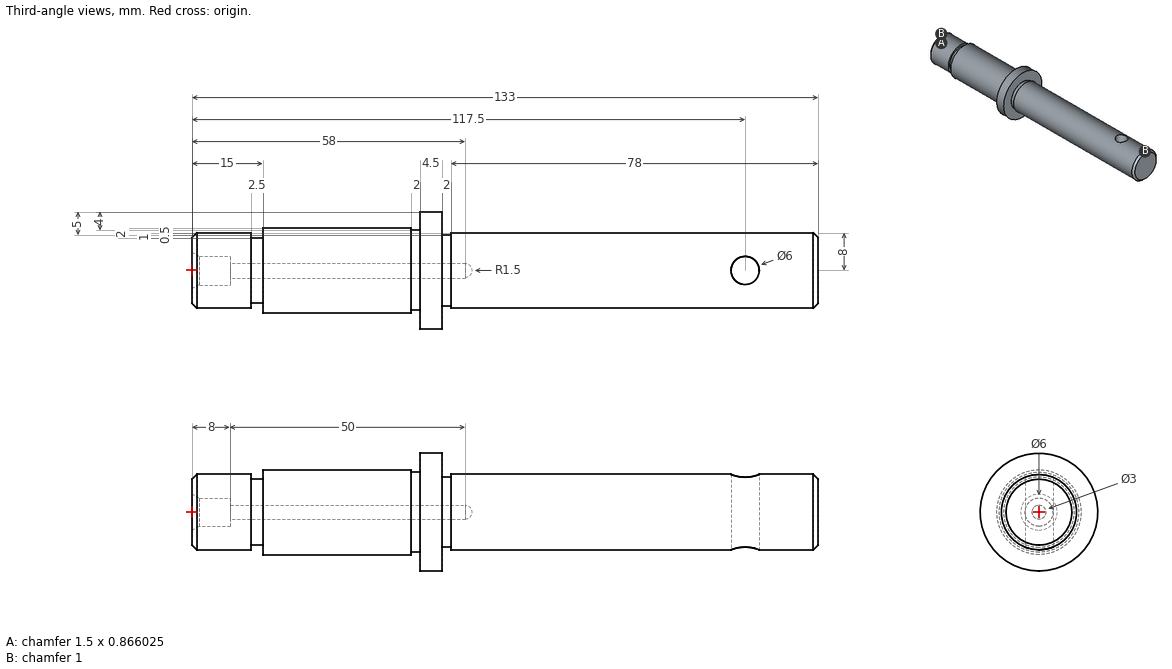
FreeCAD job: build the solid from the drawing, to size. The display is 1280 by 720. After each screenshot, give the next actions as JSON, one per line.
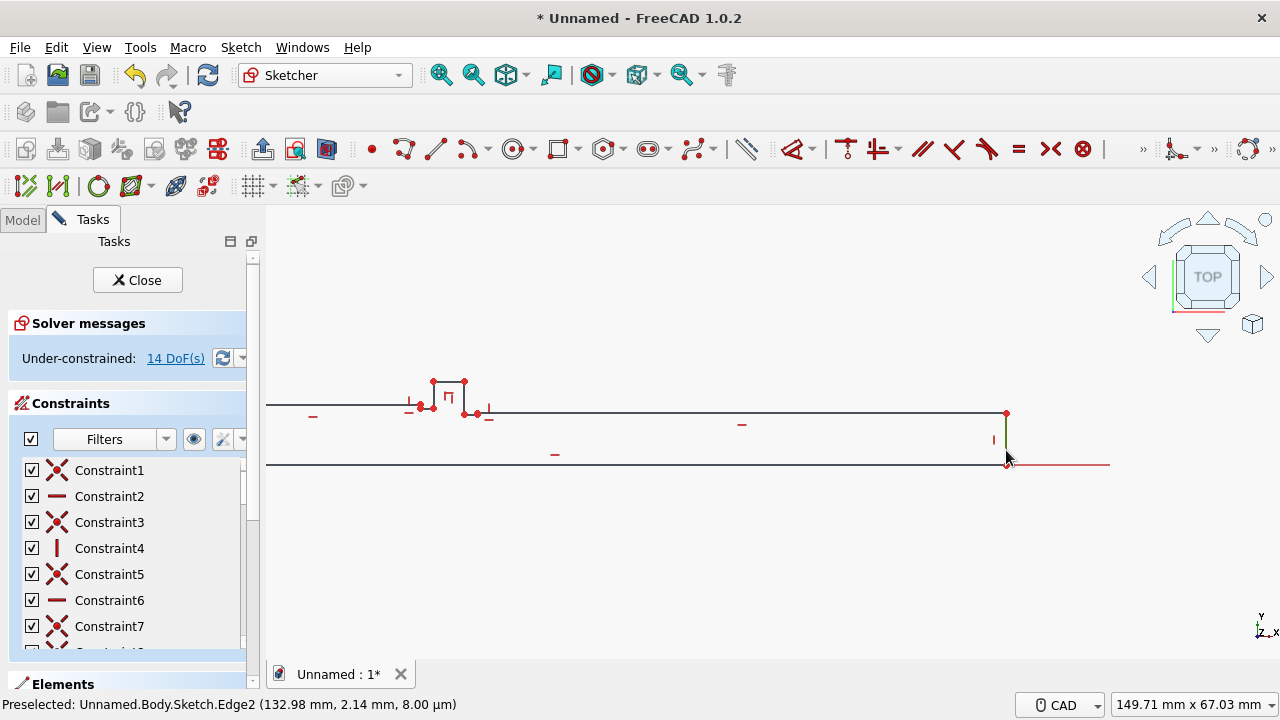
{"action": "left_click", "coordinate": [814, 150]}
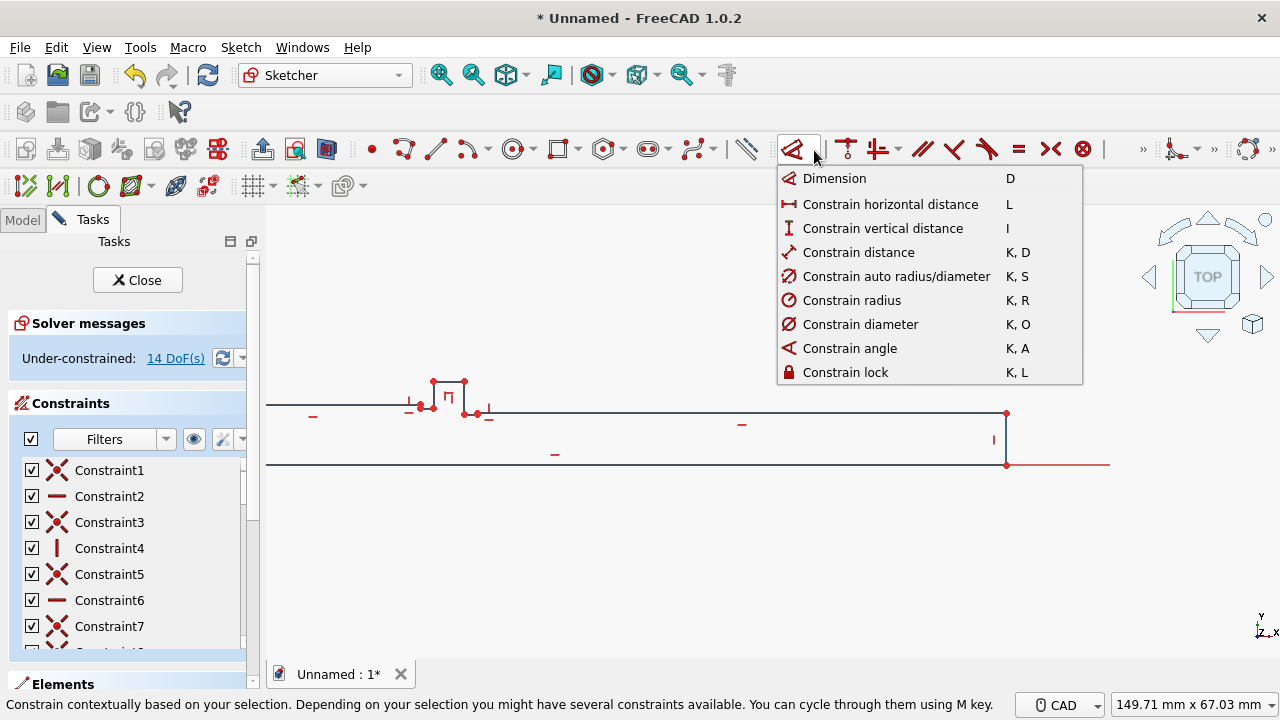
{"action": "left_click", "coordinate": [930, 228]}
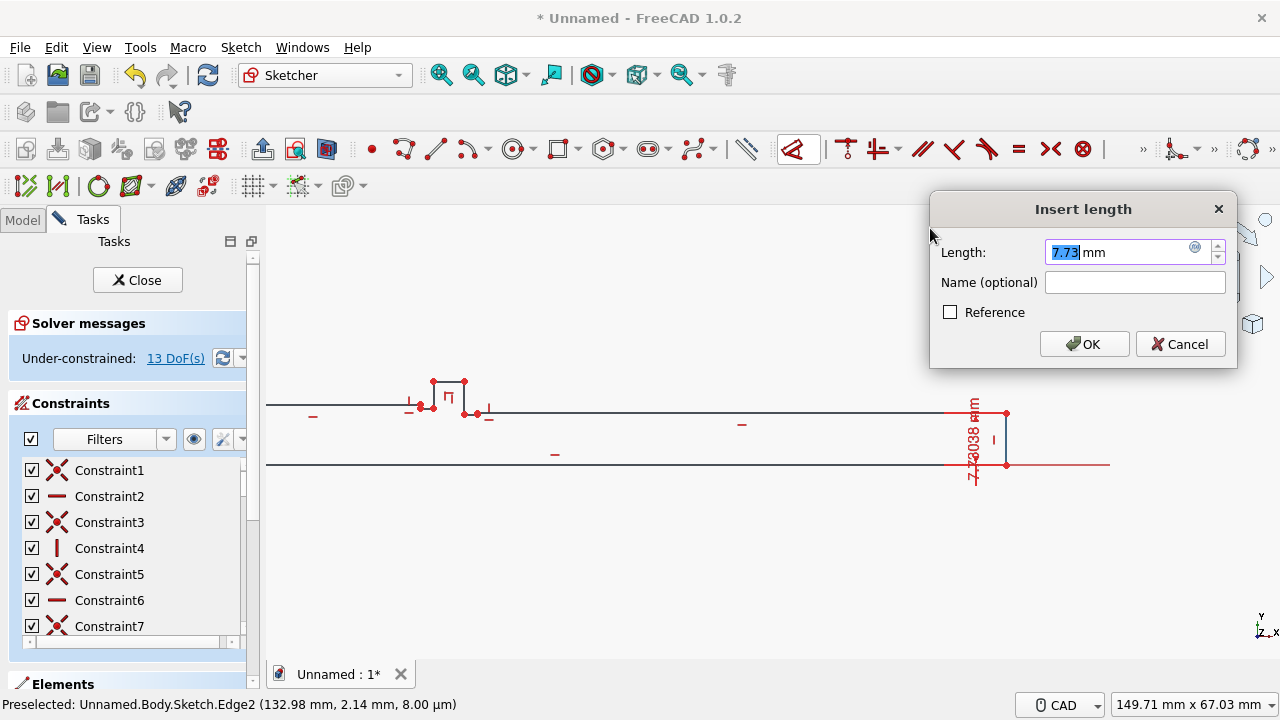
{"action": "type", "text": "8"}
{"action": "key", "text": "Return"}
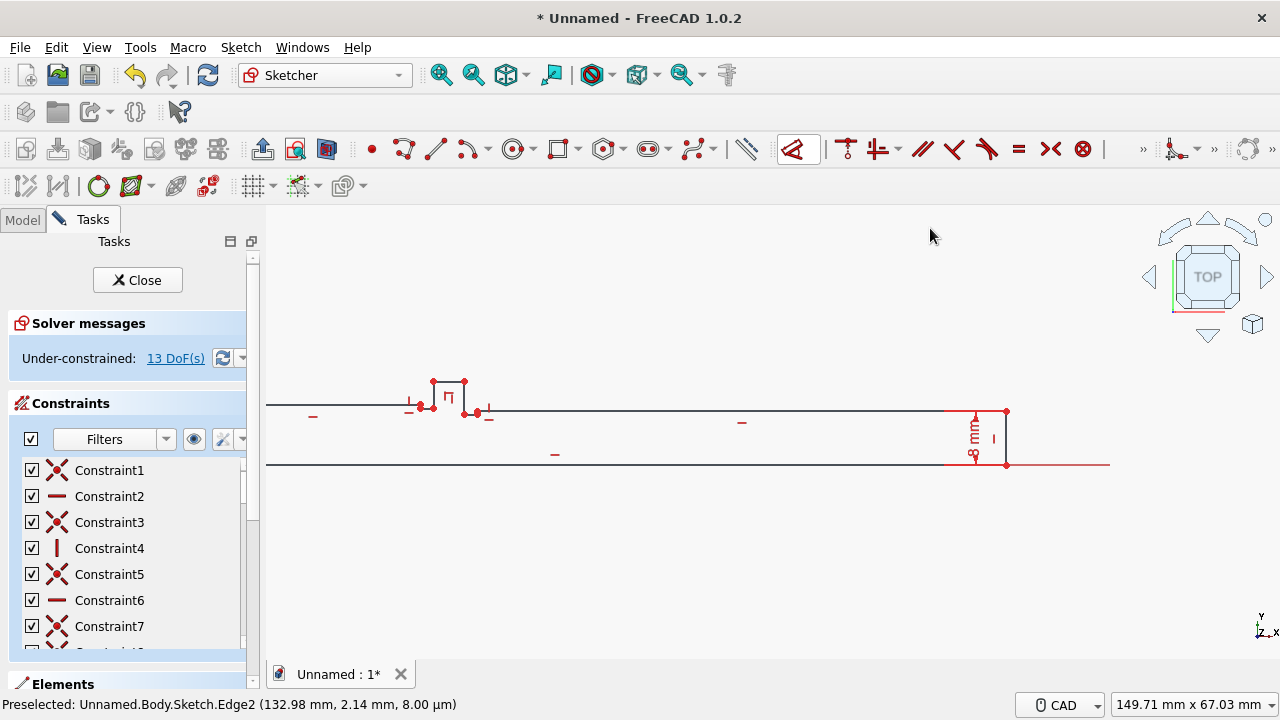
{"action": "scroll", "coordinate": [471, 415], "scroll_direction": "up", "scroll_amount": 6}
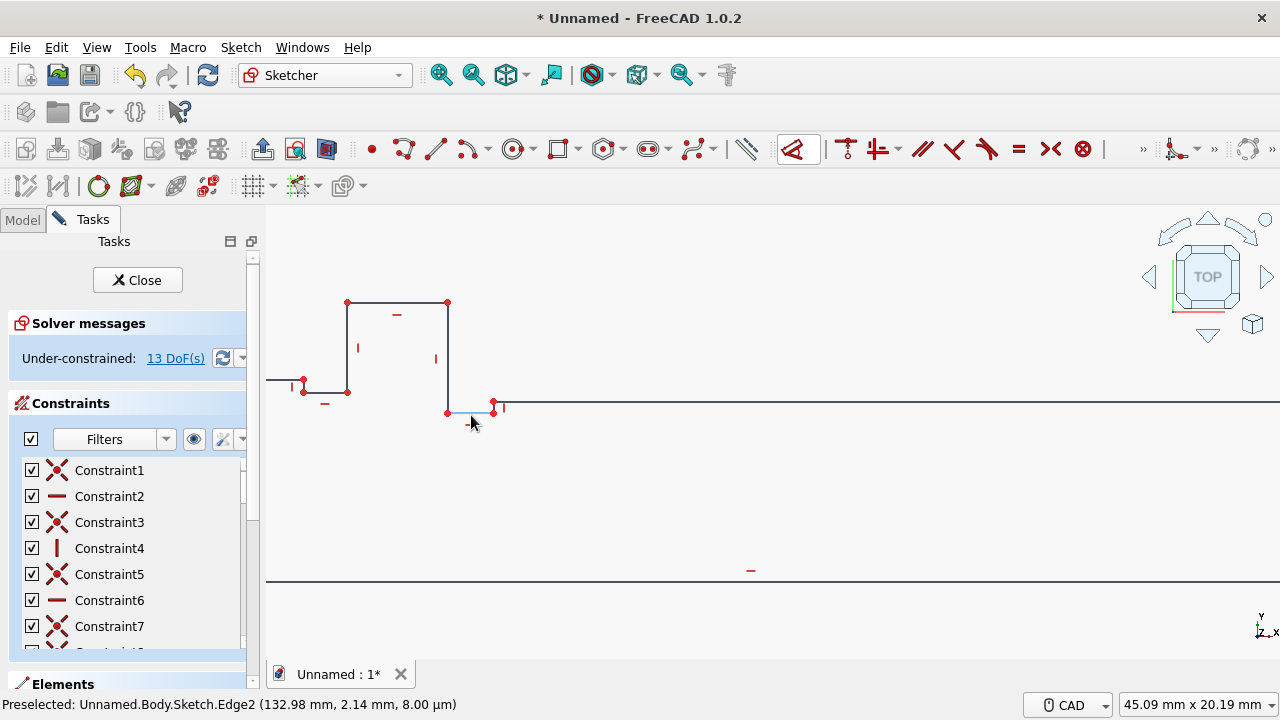
{"action": "left_click", "coordinate": [471, 413]}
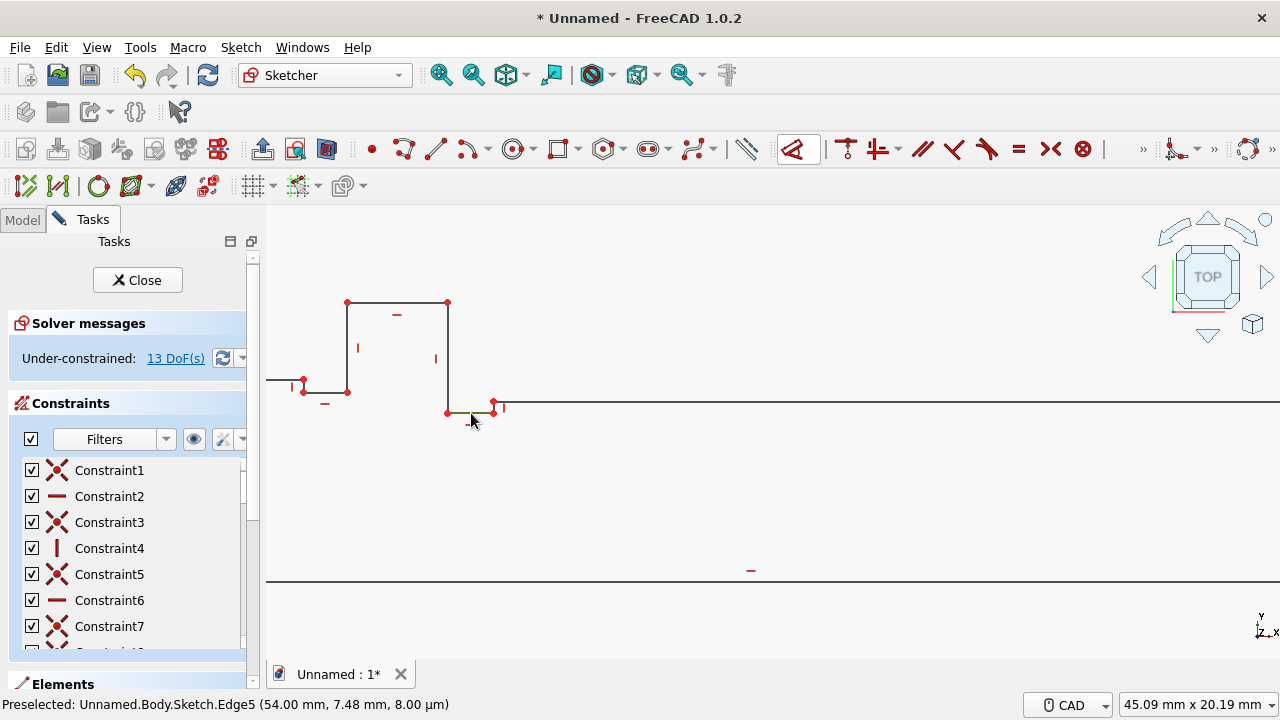
{"action": "key", "text": "l"}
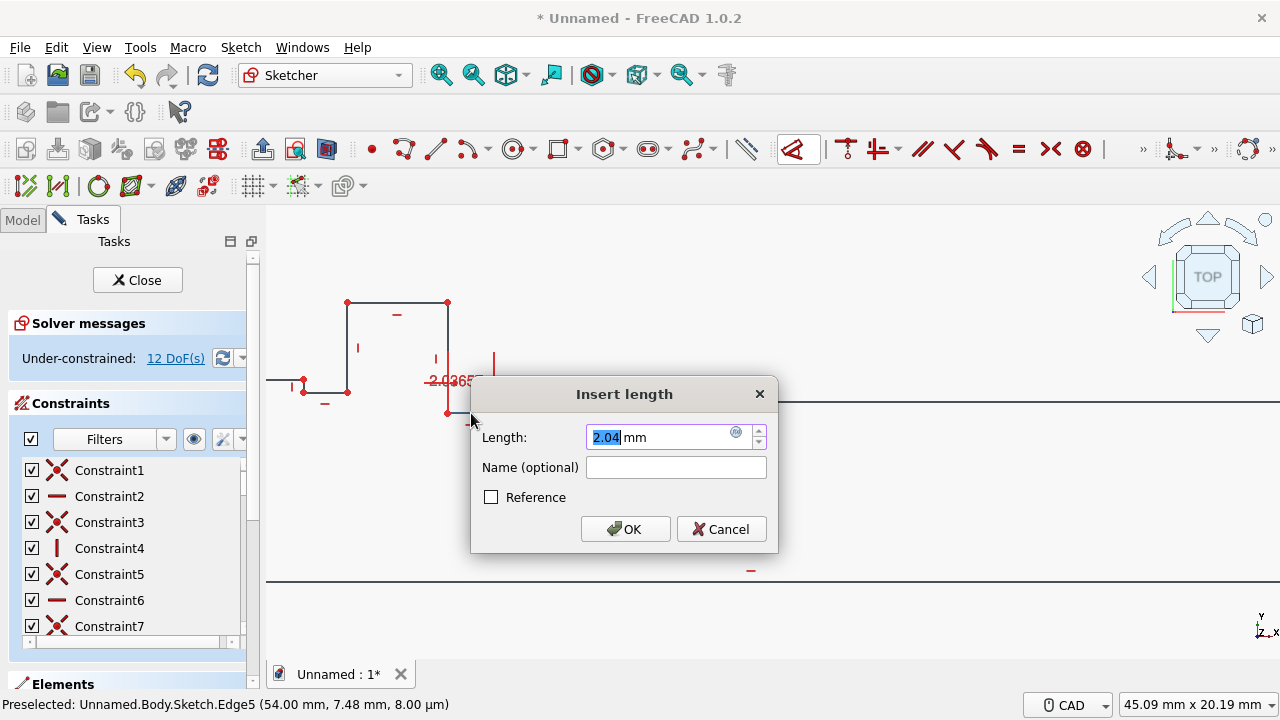
{"action": "type", "text": "2"}
{"action": "key", "text": "Return"}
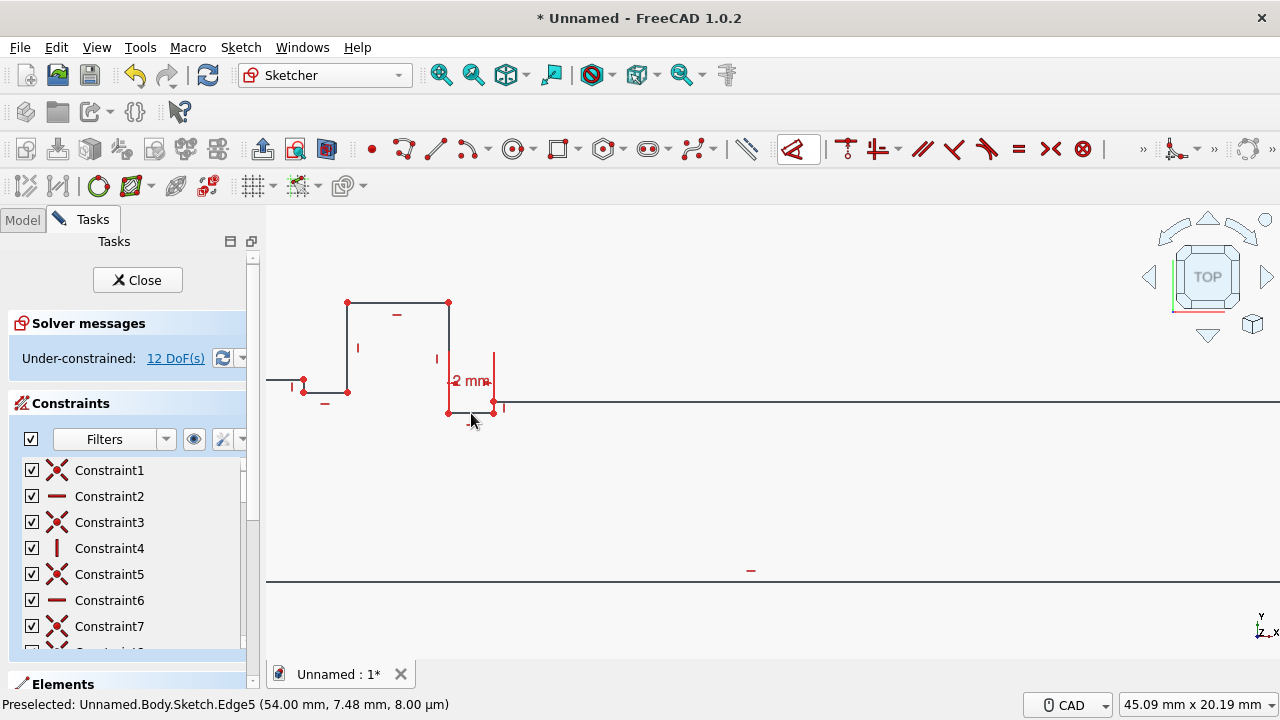
{"action": "left_click", "coordinate": [449, 380]}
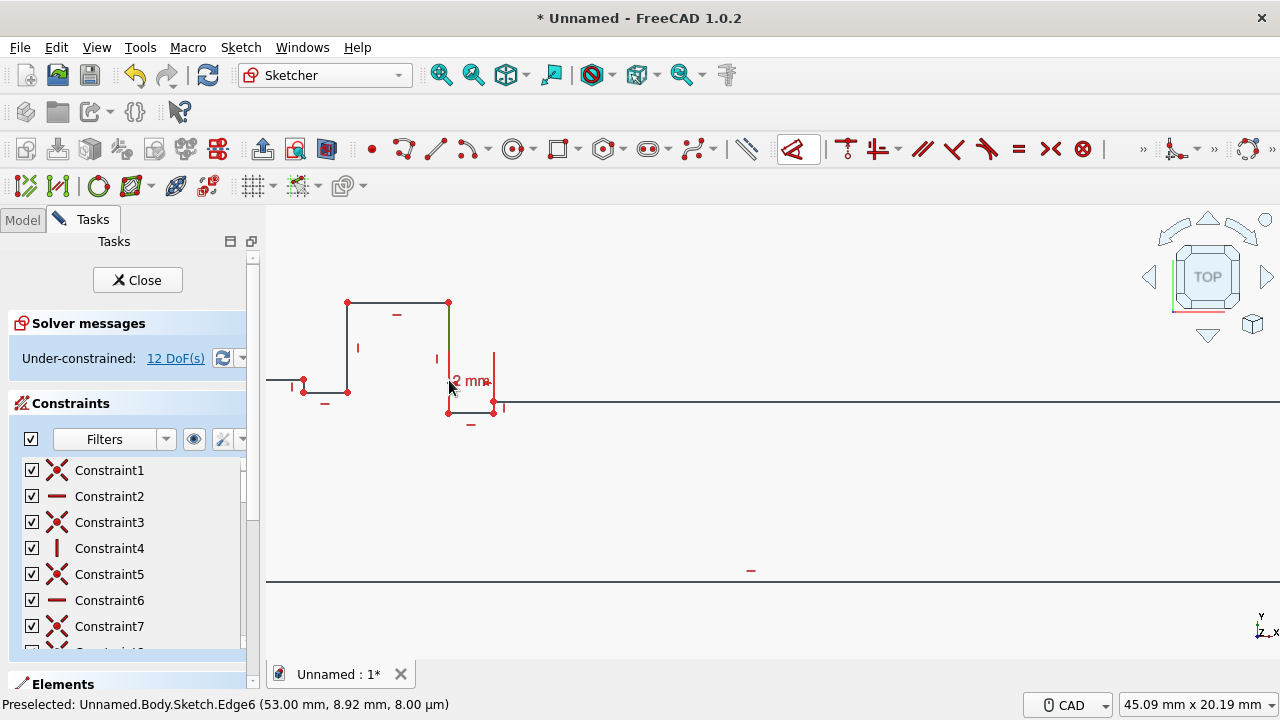
{"action": "left_click", "coordinate": [814, 150]}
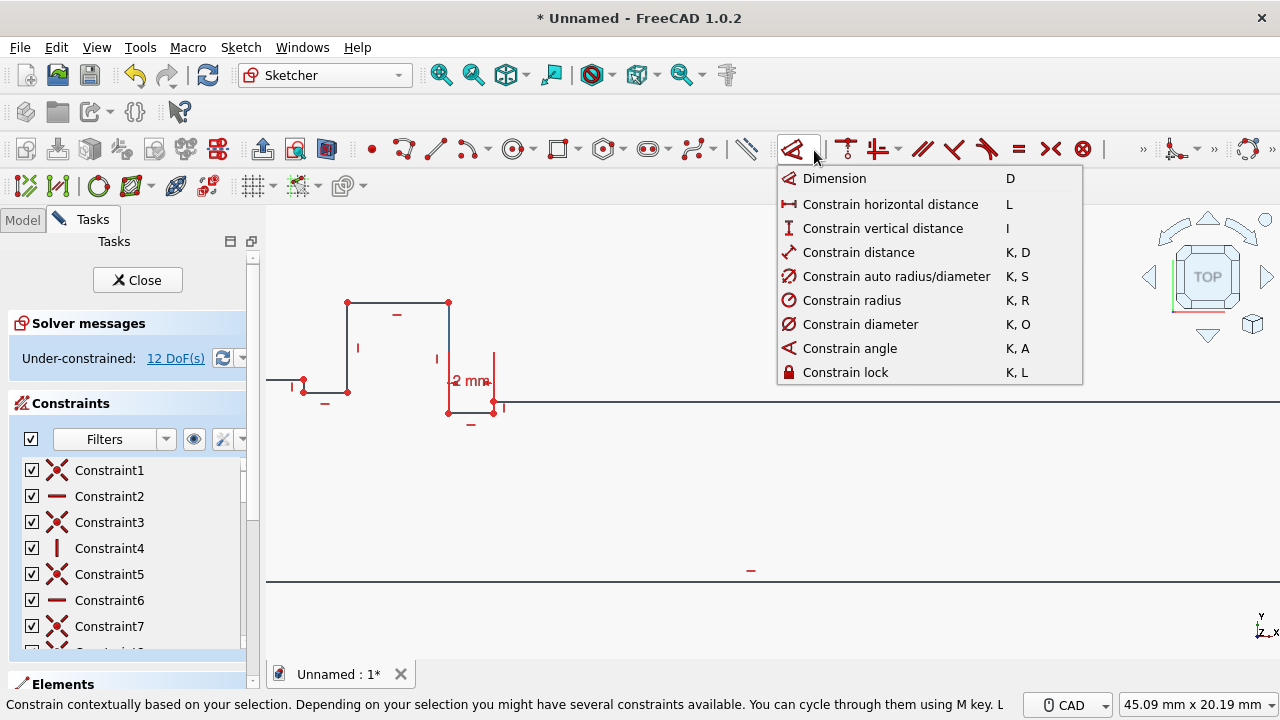
{"action": "left_click", "coordinate": [930, 228]}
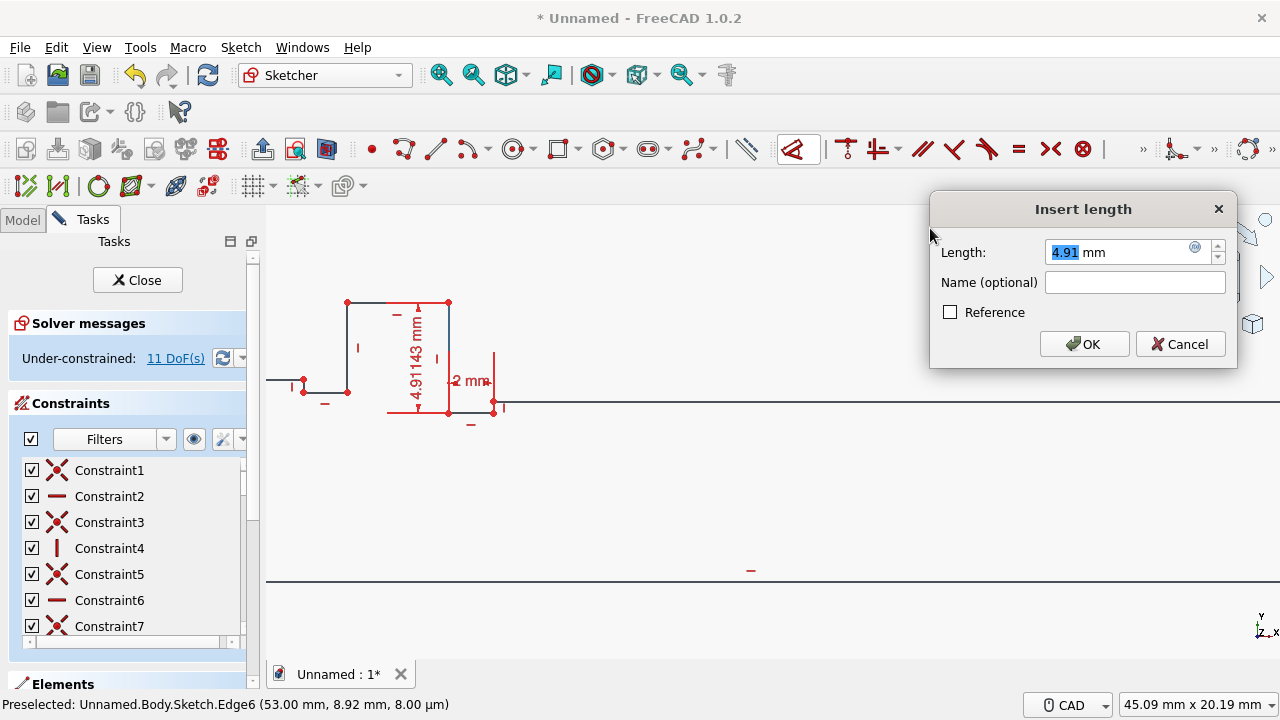
{"action": "type", "text": "5"}
{"action": "key", "text": "Return"}